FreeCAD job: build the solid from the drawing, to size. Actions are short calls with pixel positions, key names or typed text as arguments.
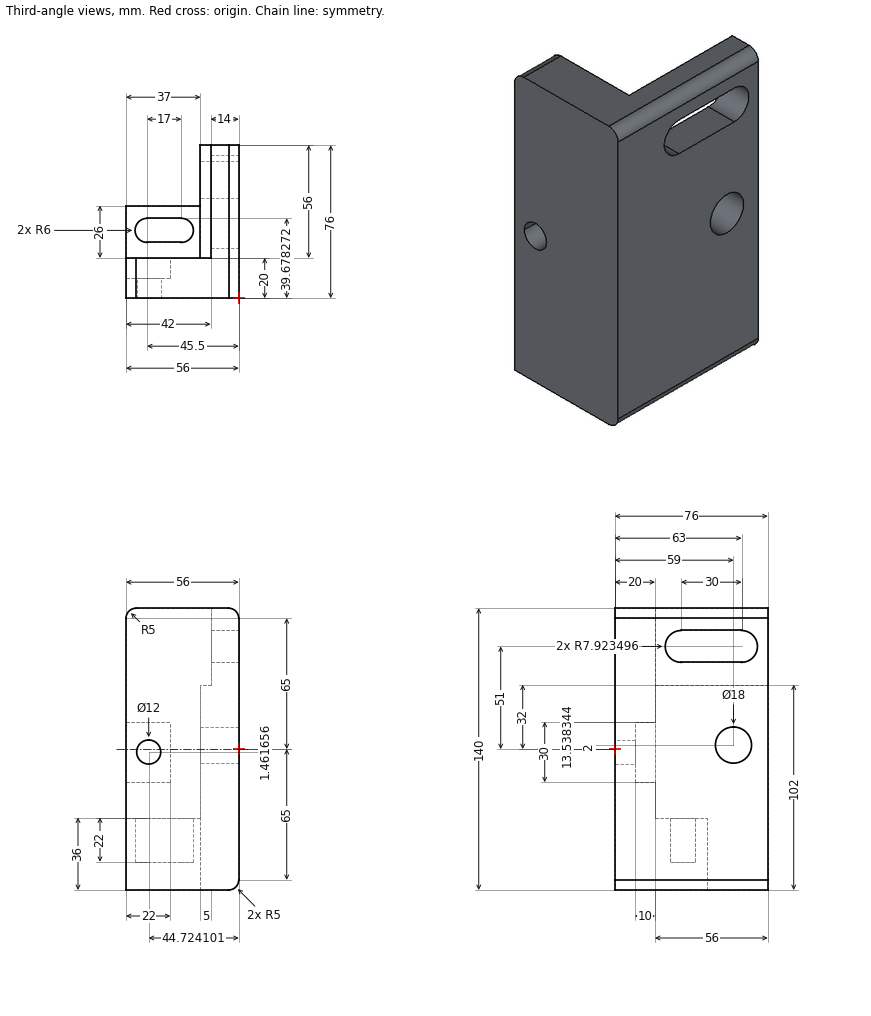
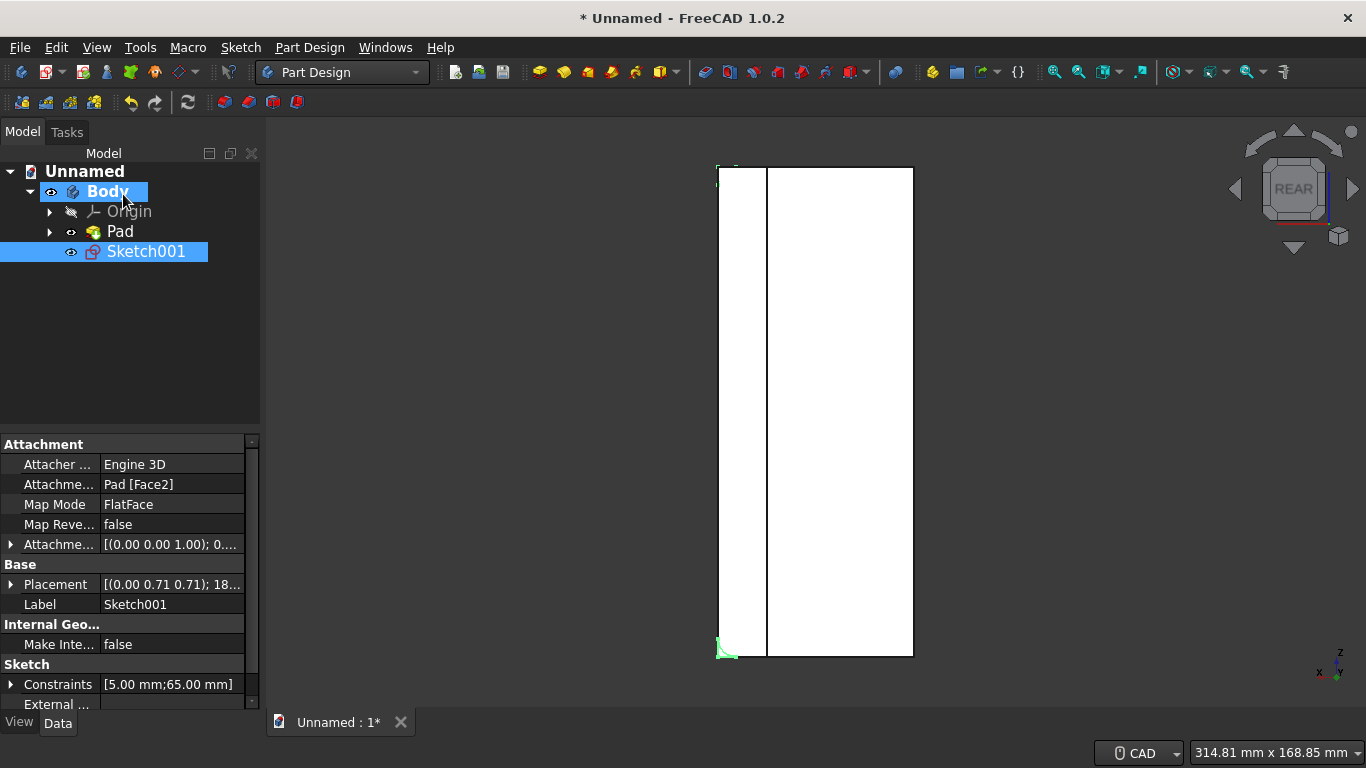
click(706, 72)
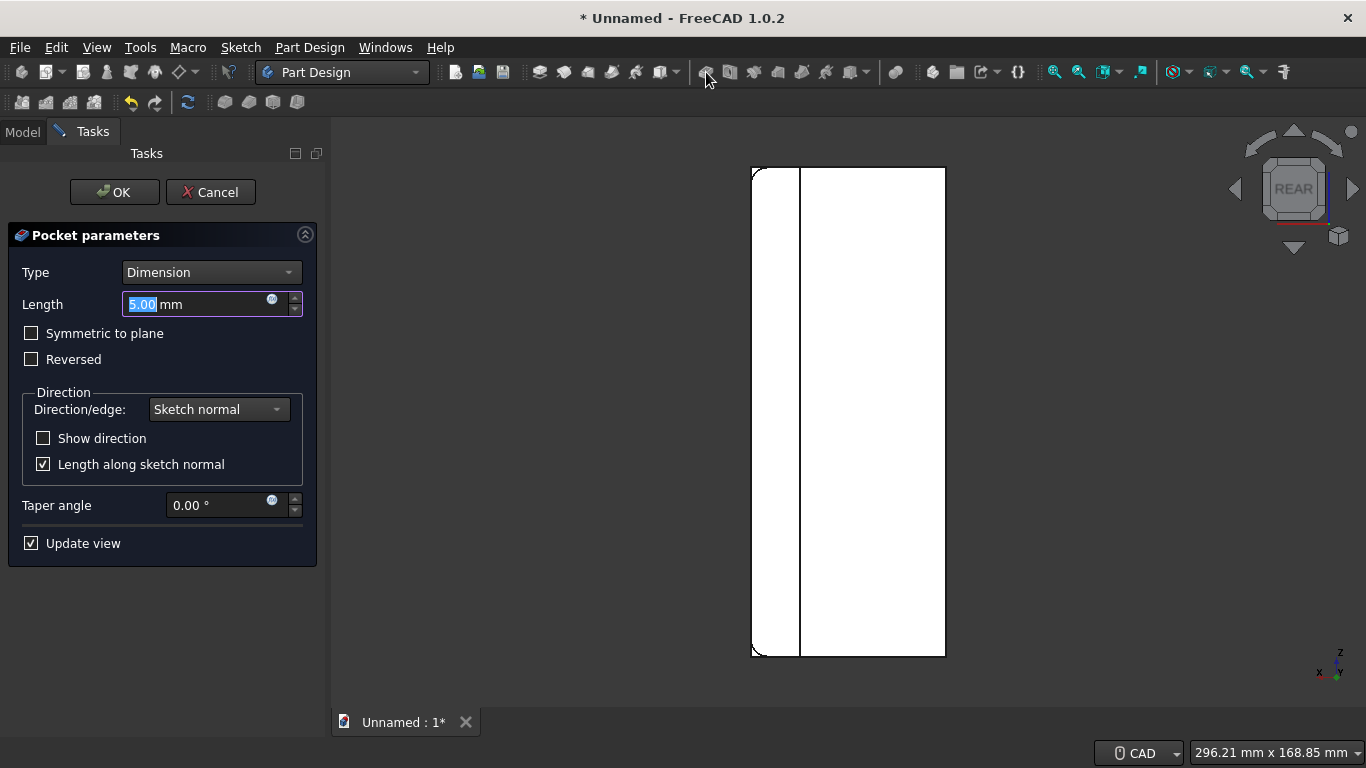
click(212, 272)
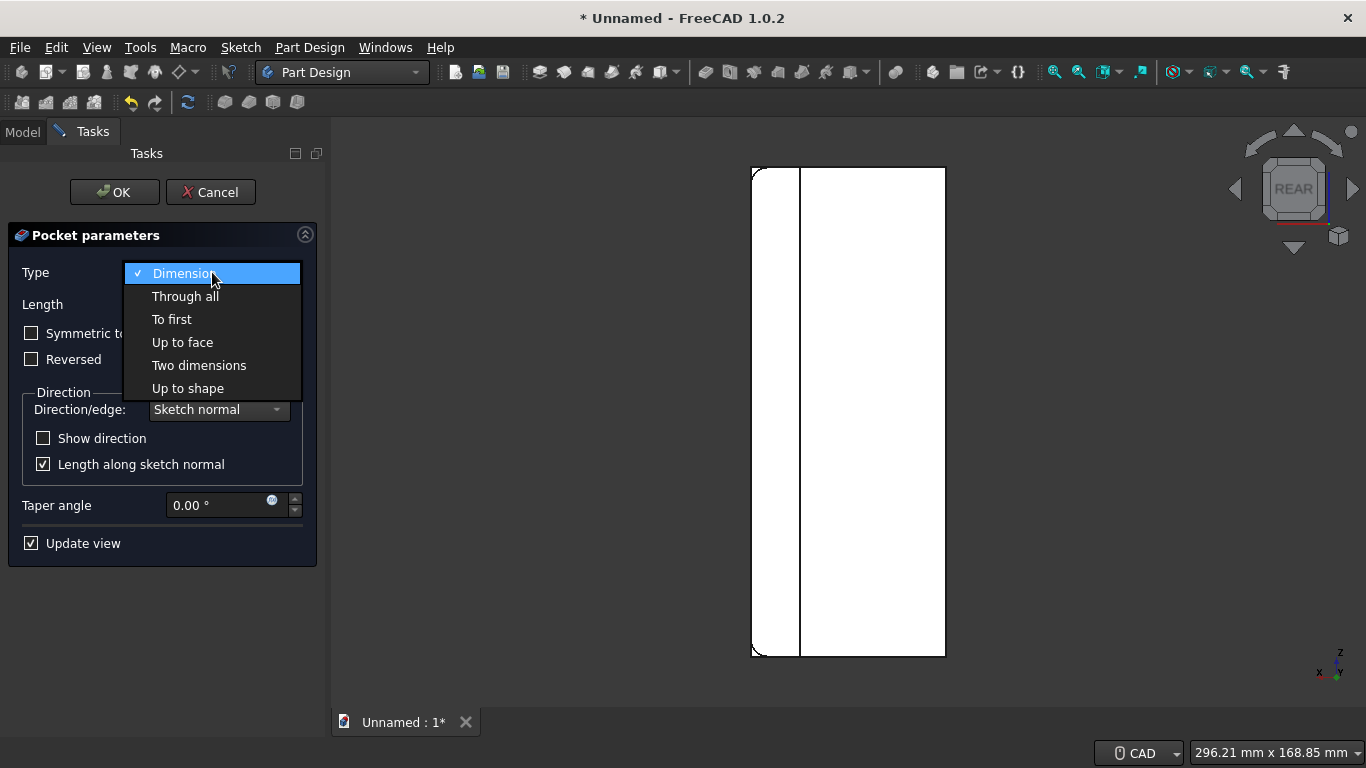
click(212, 296)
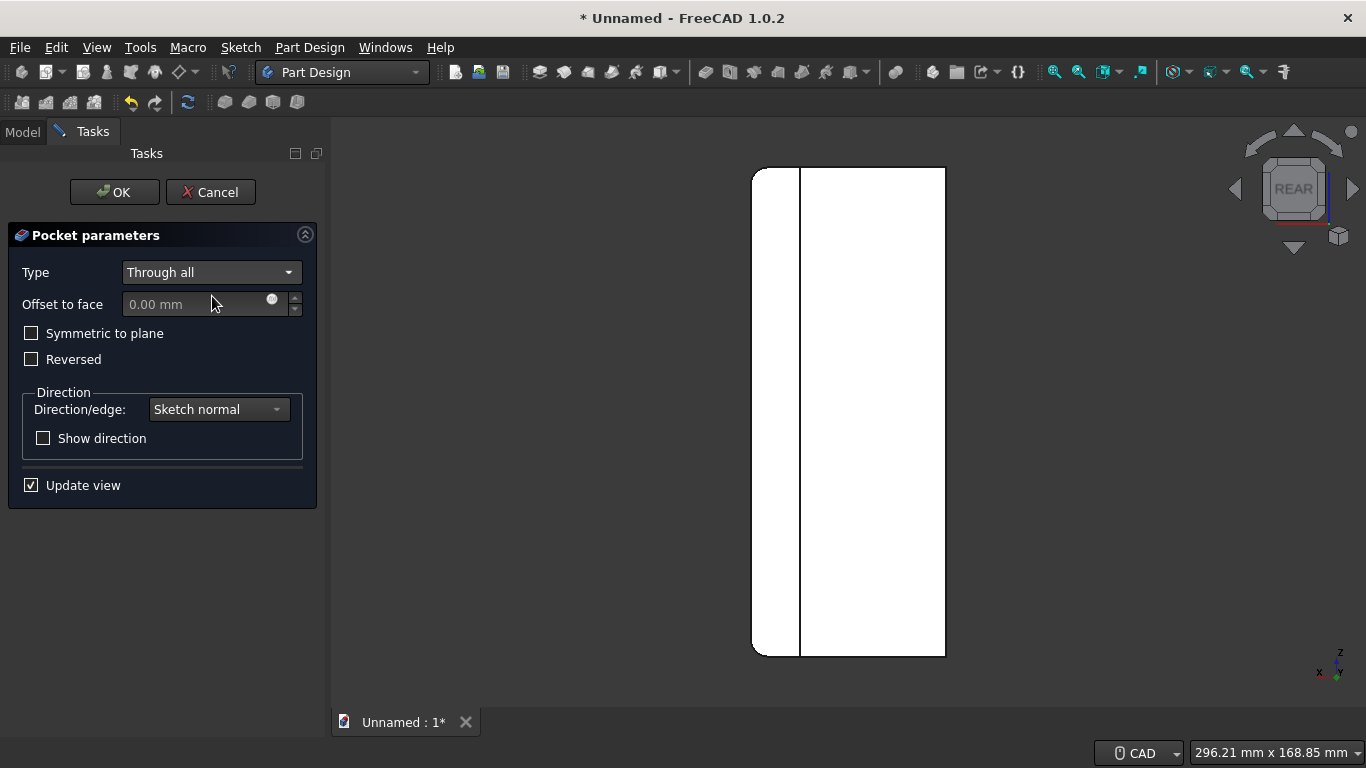
click(115, 192)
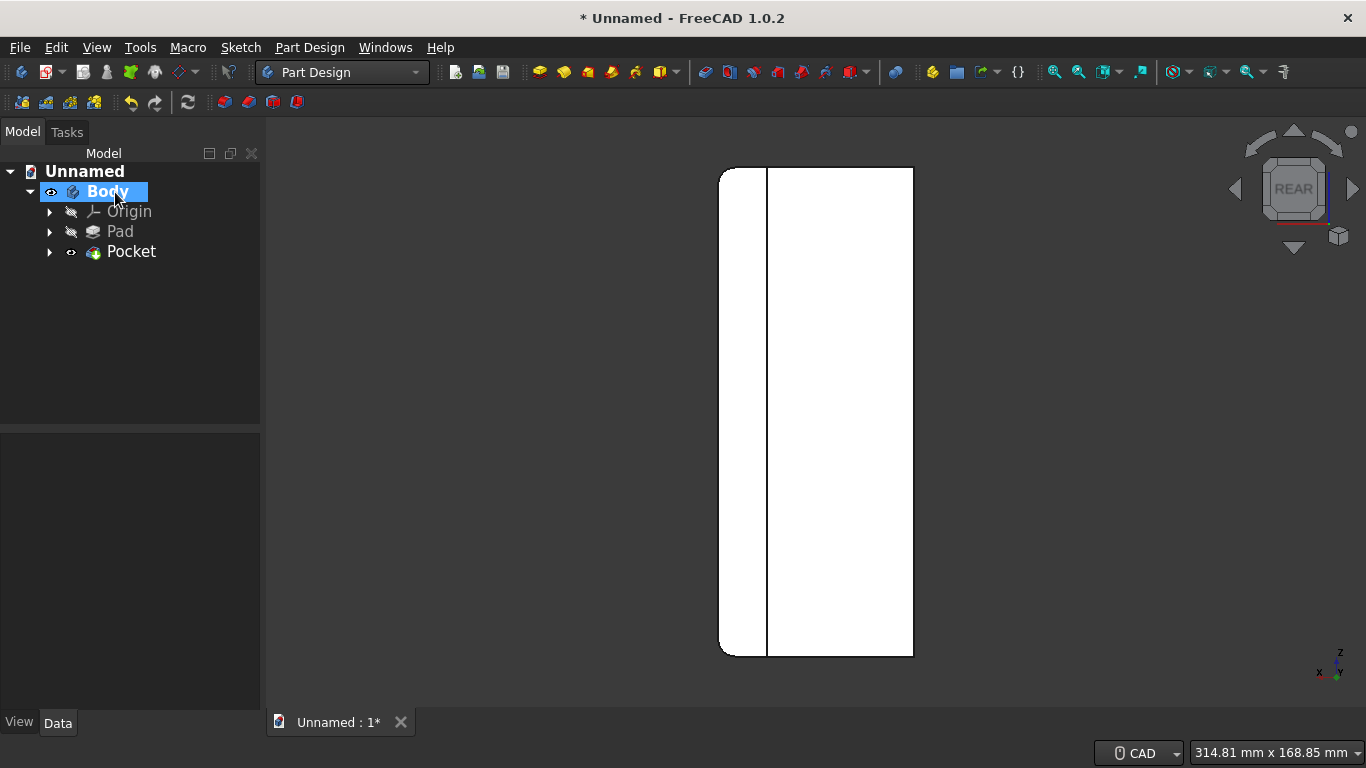
click(840, 271)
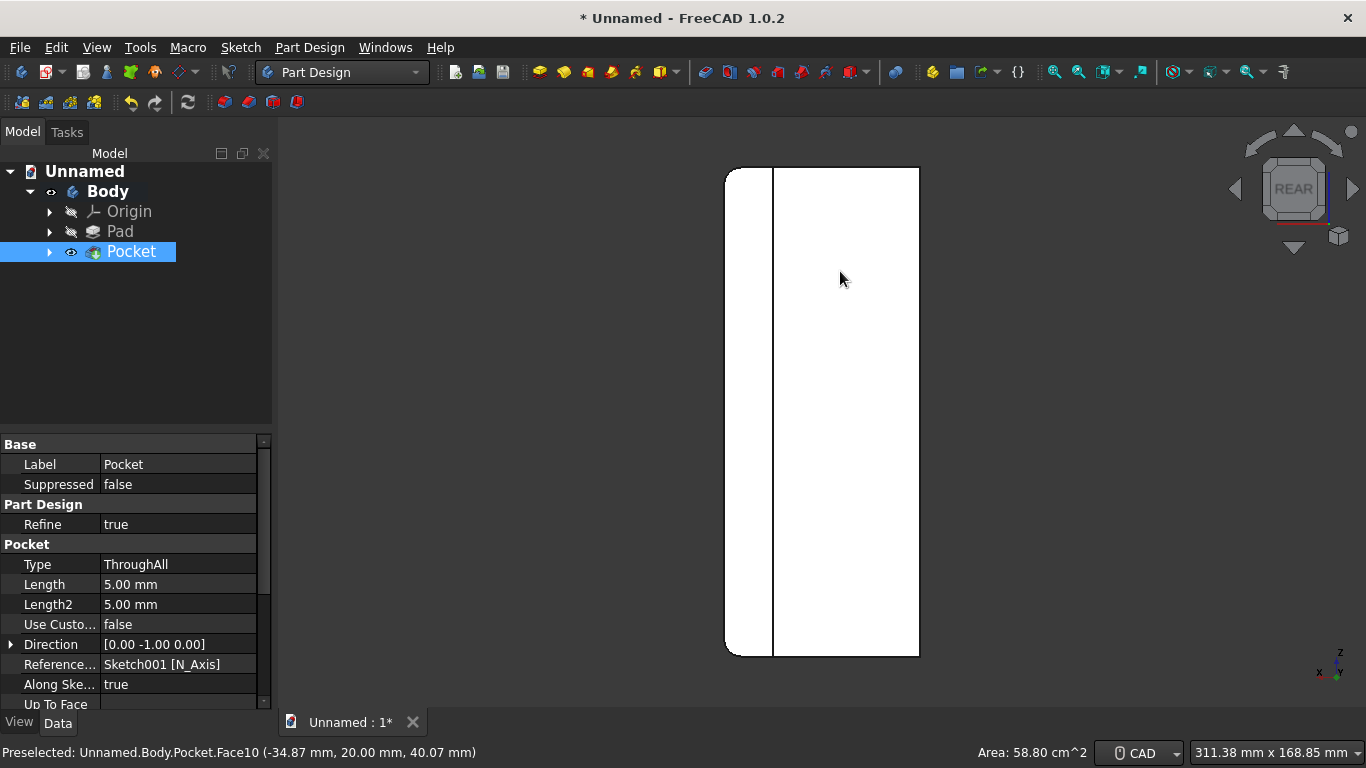
click(46, 72)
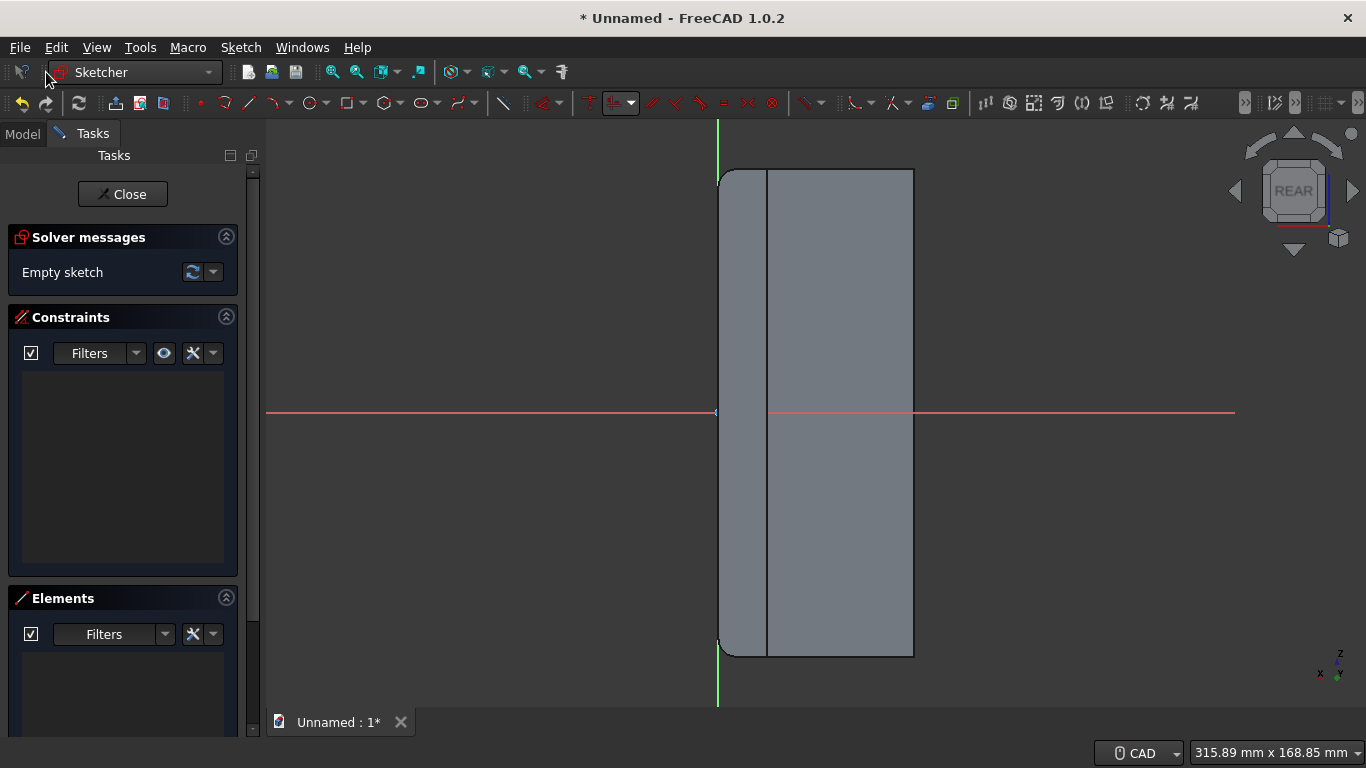
click(164, 104)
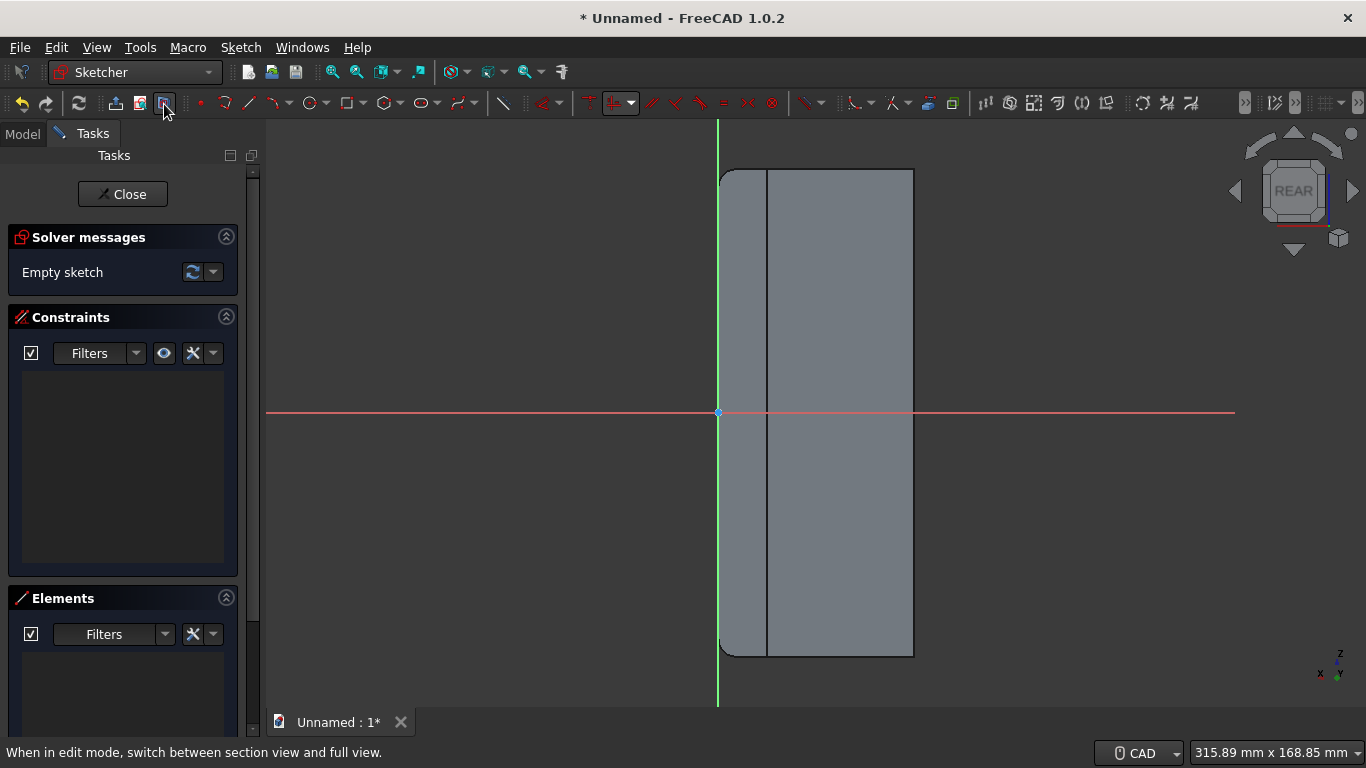
scroll(913, 166, up, 15)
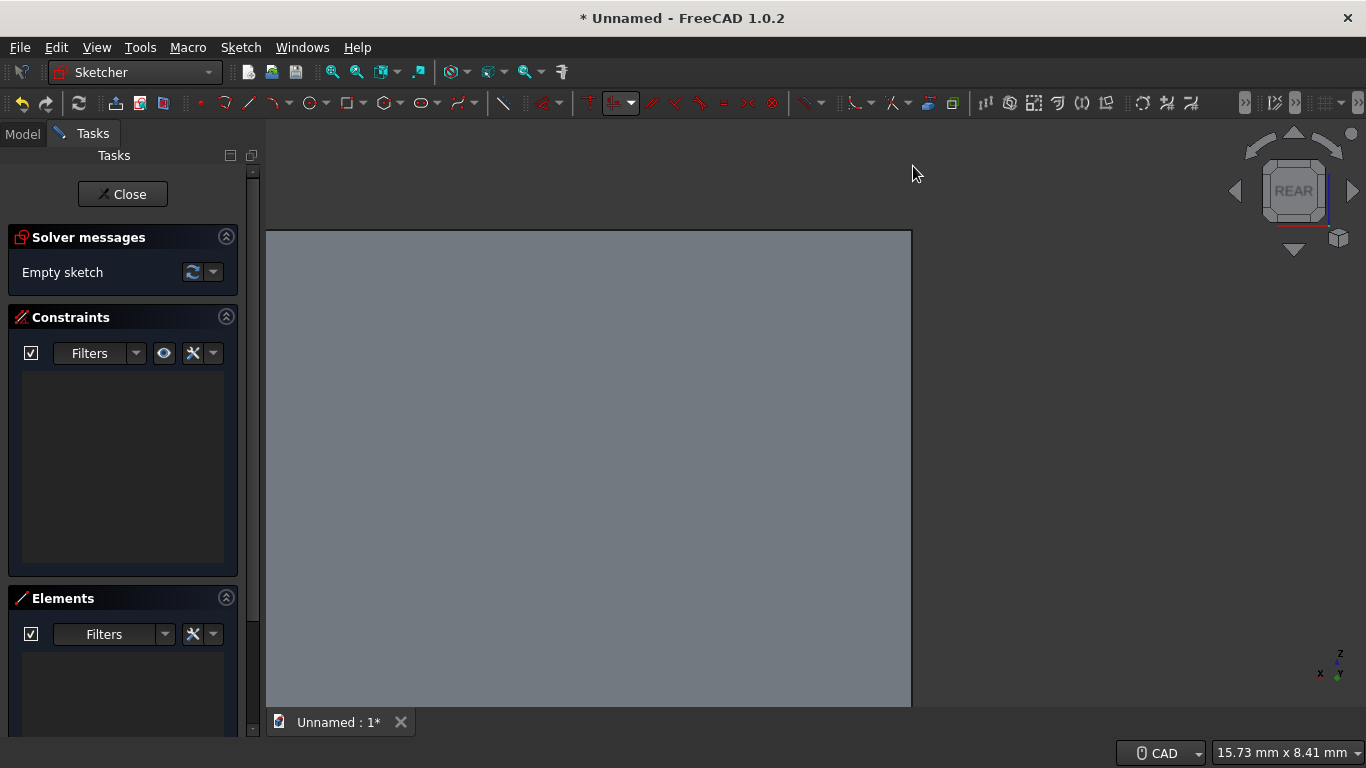
click(226, 104)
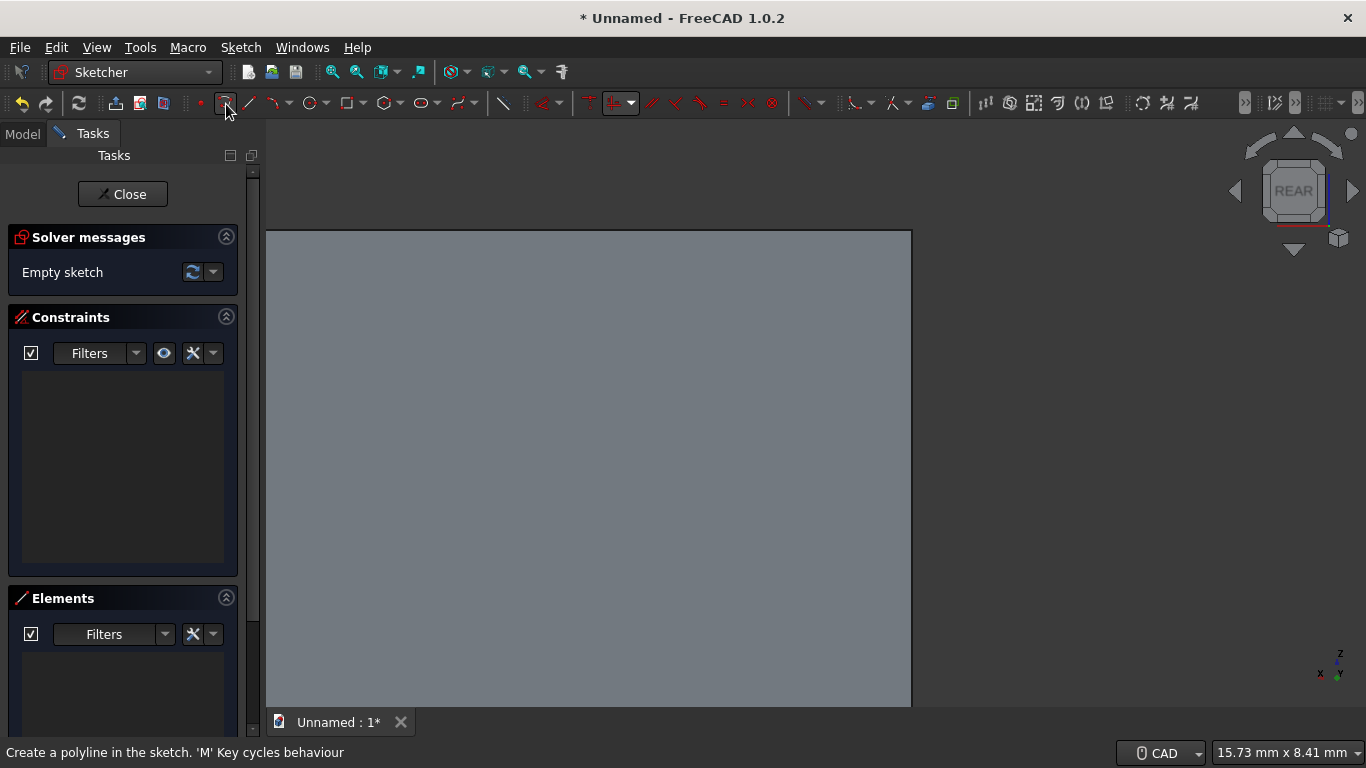
click(912, 579)
click(912, 230)
click(562, 230)
right_click(562, 230)